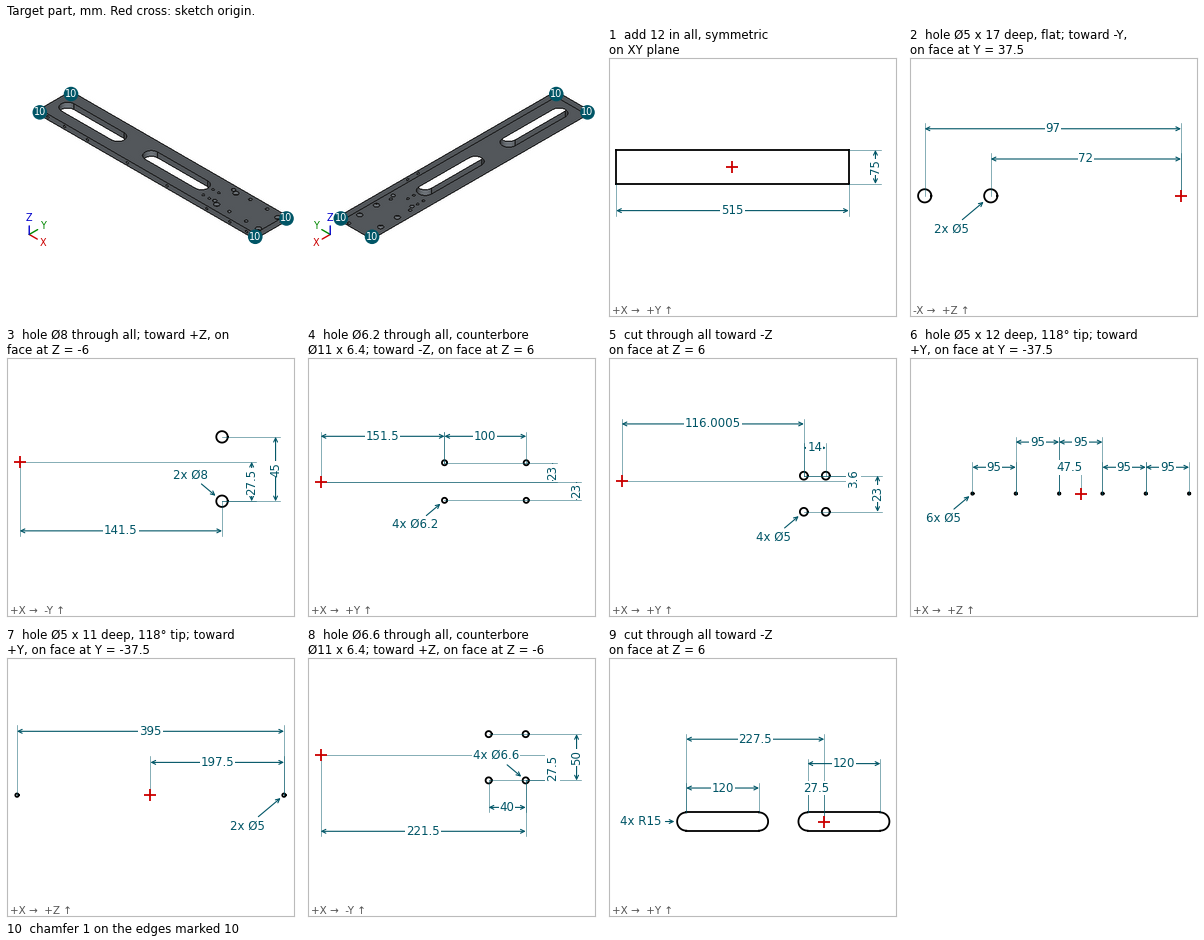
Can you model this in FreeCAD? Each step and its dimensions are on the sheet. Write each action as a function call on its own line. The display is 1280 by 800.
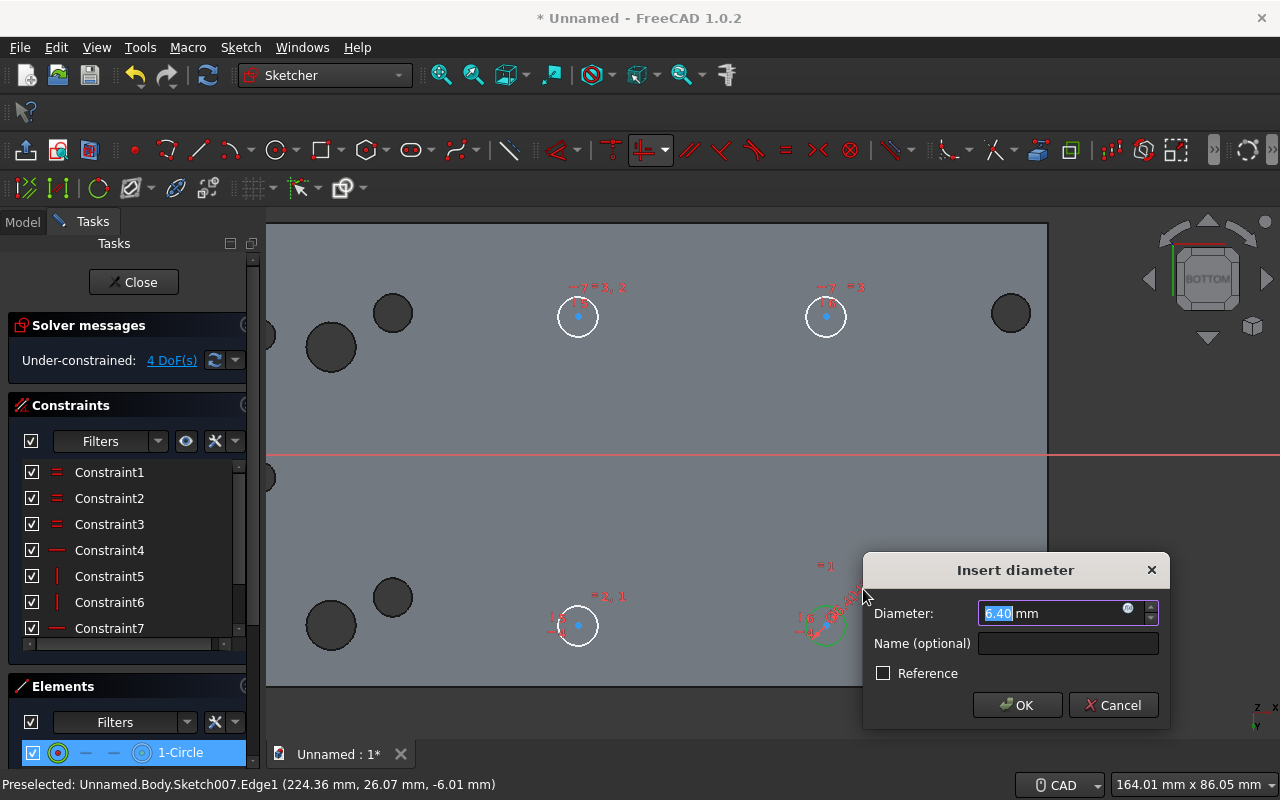
text(6.6)
key(Return)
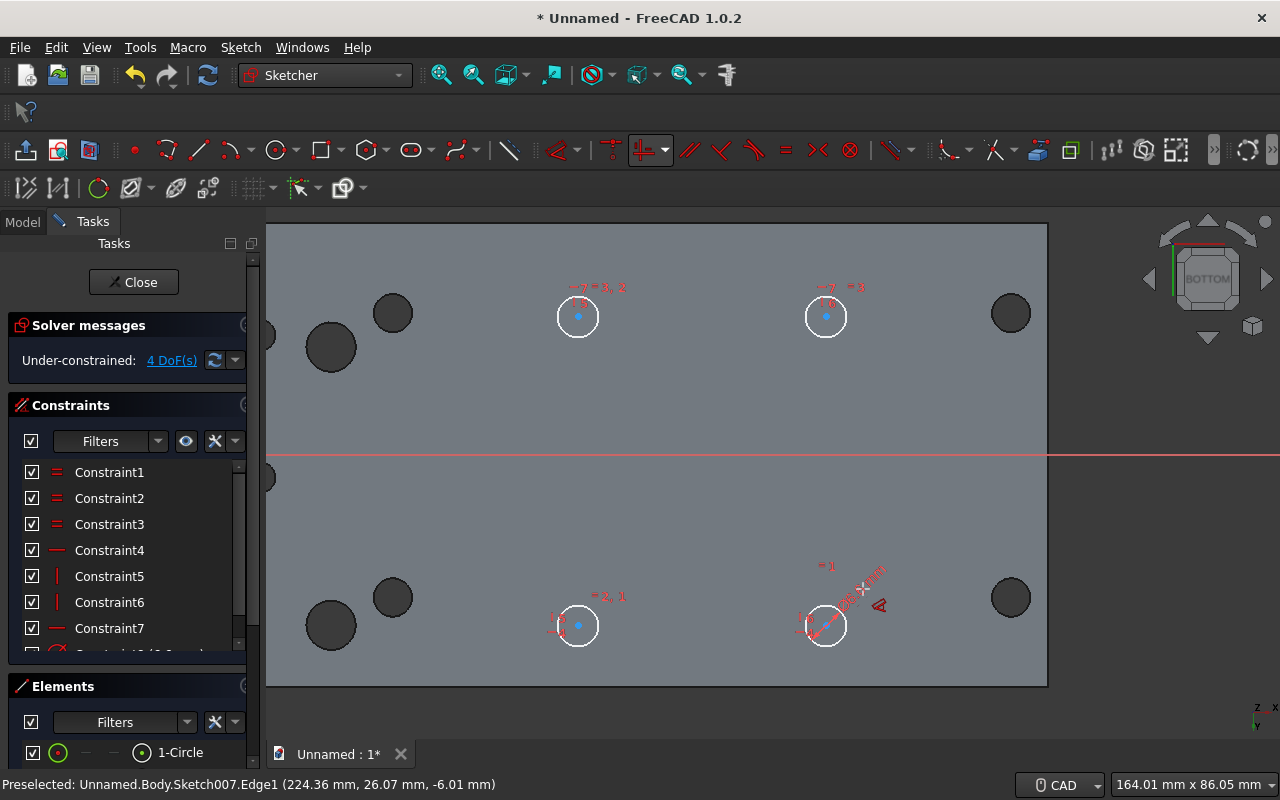
click(826, 626)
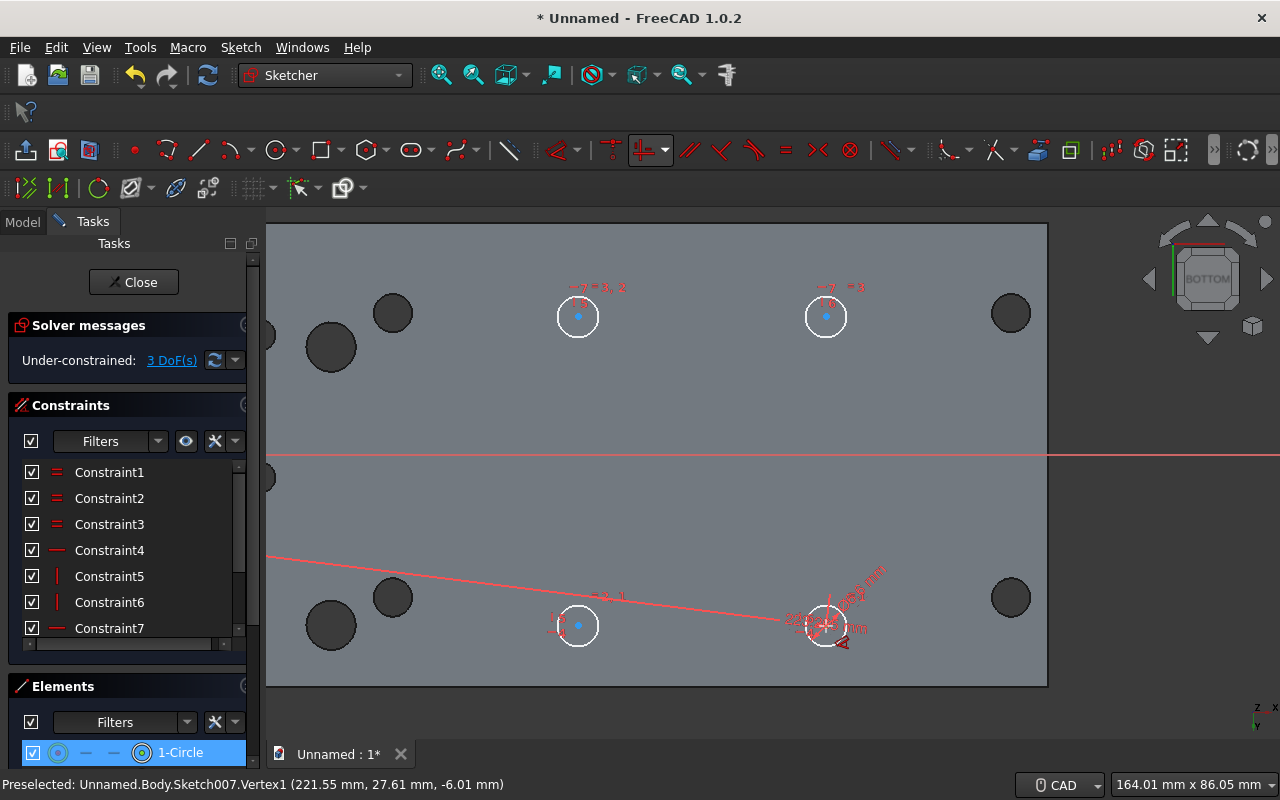
click(578, 626)
click(702, 660)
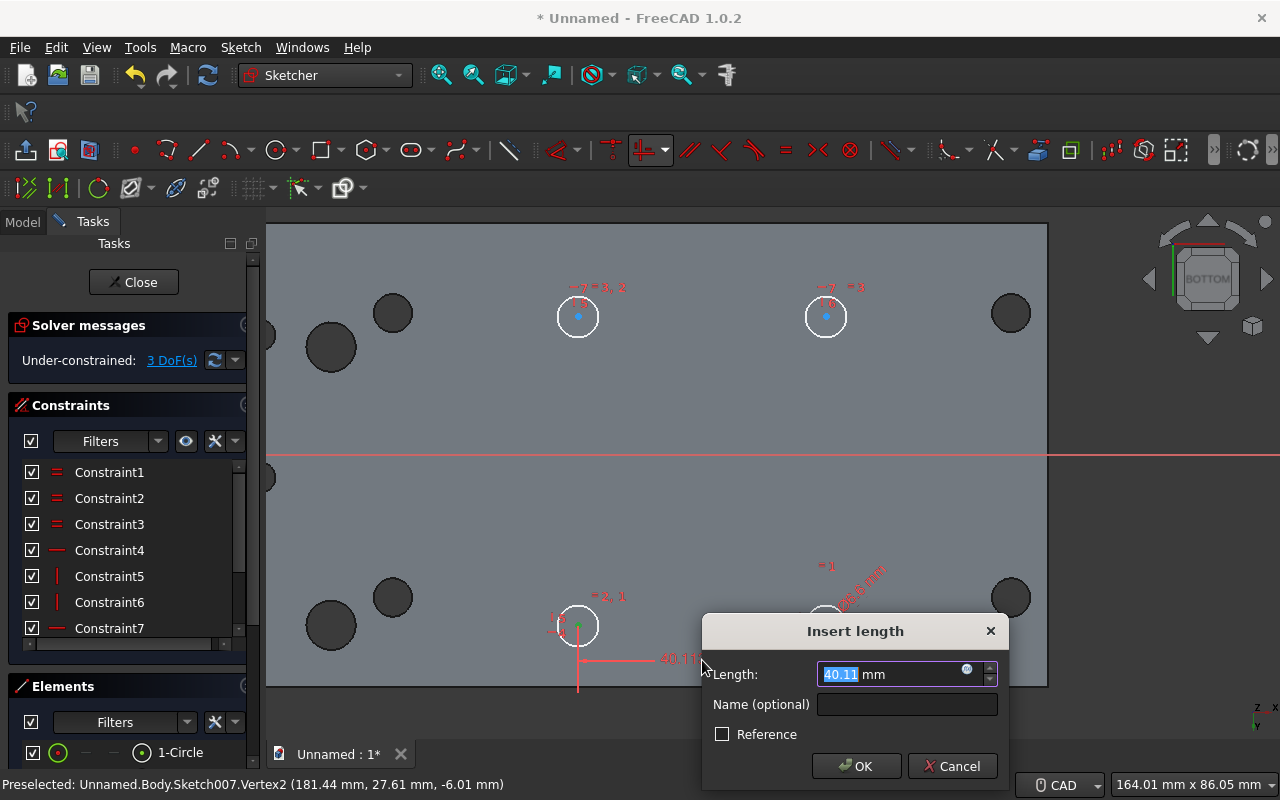
text(40)
key(Return)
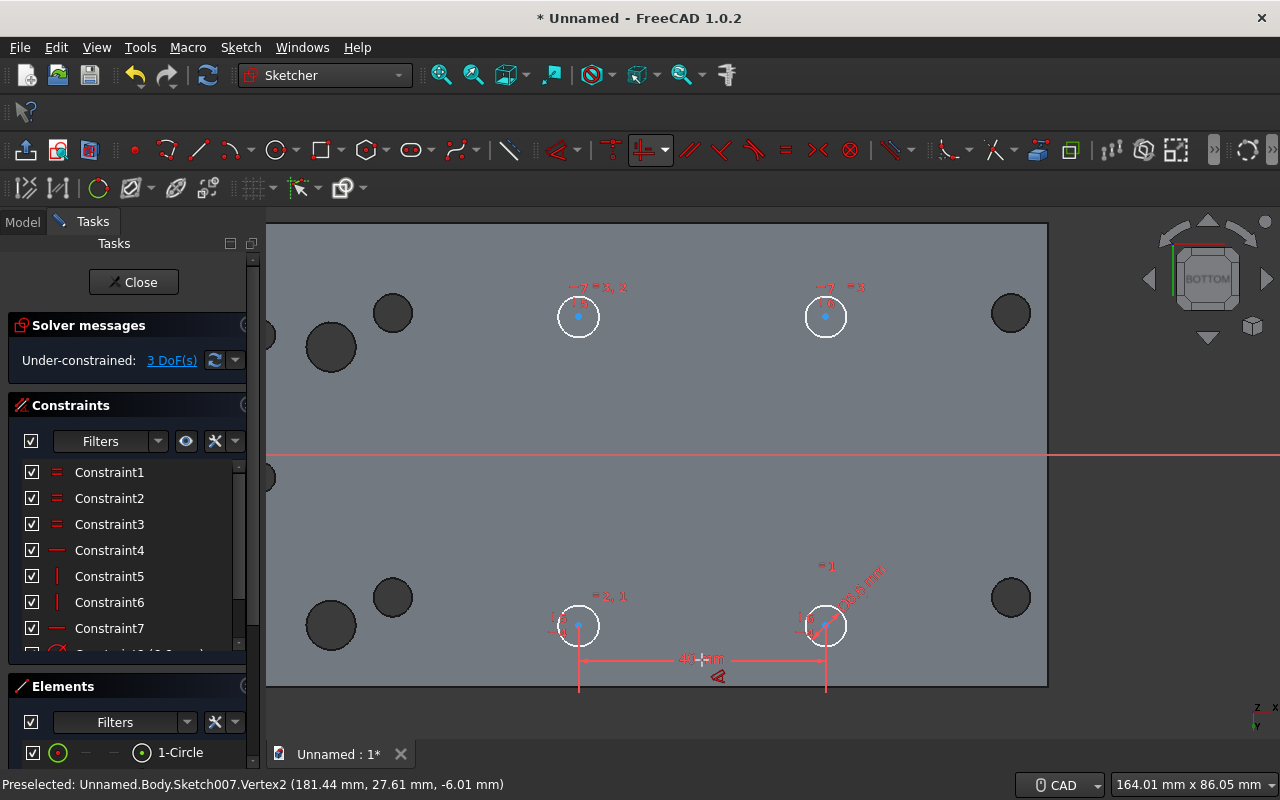
click(579, 626)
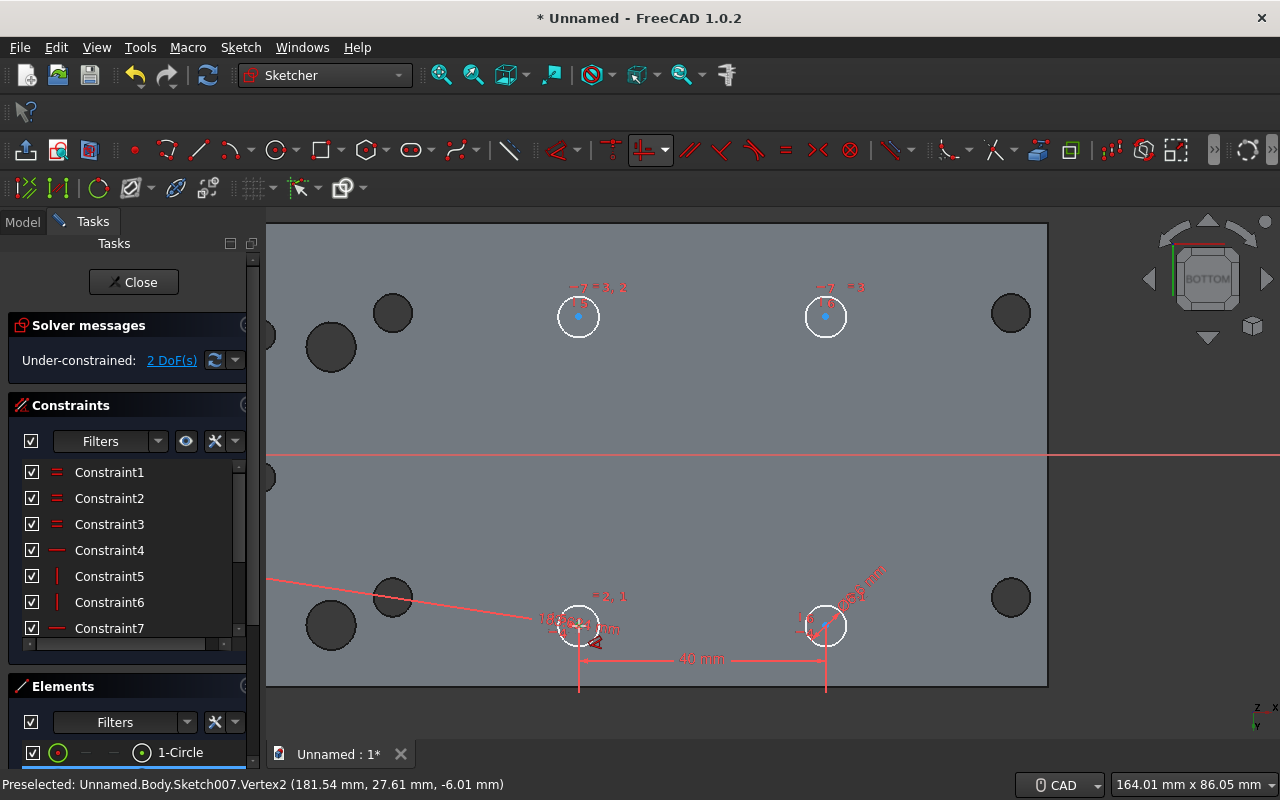
click(579, 317)
click(545, 471)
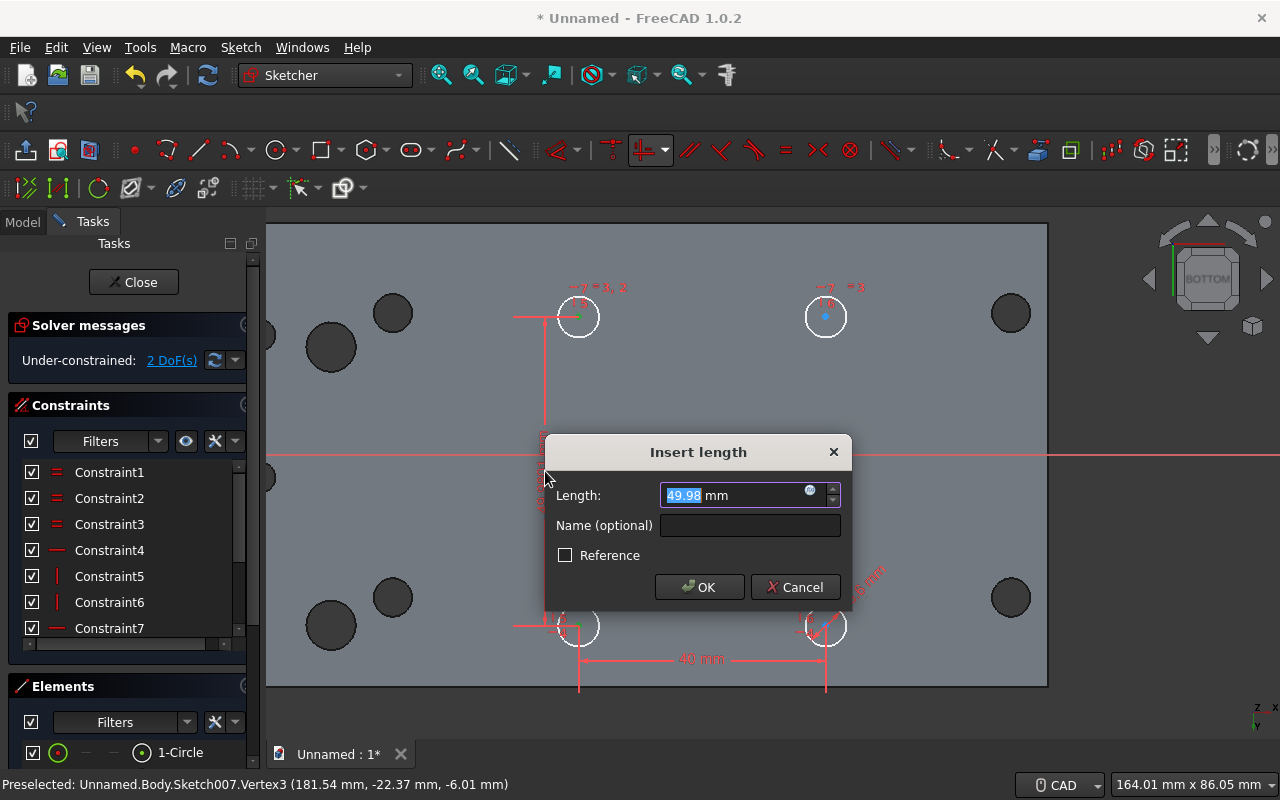
text(50)
key(Return)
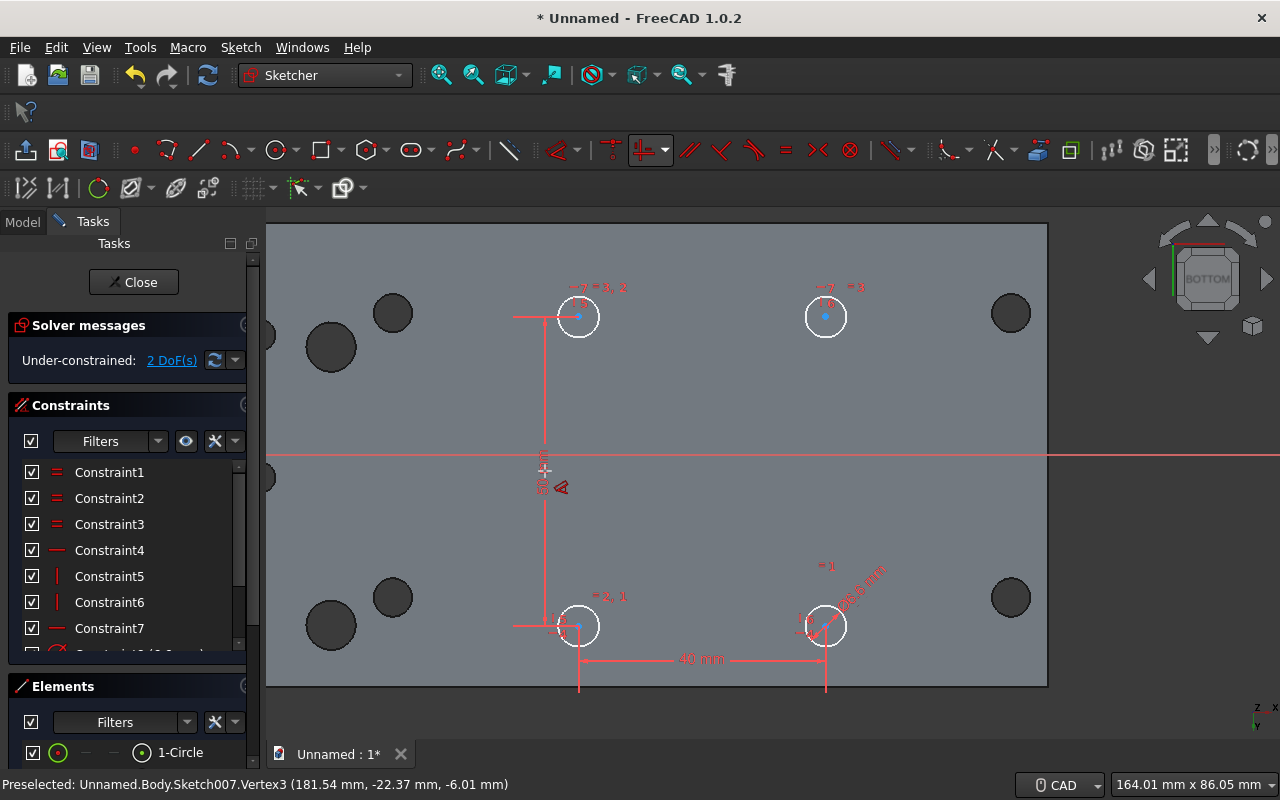
click(826, 626)
click(860, 541)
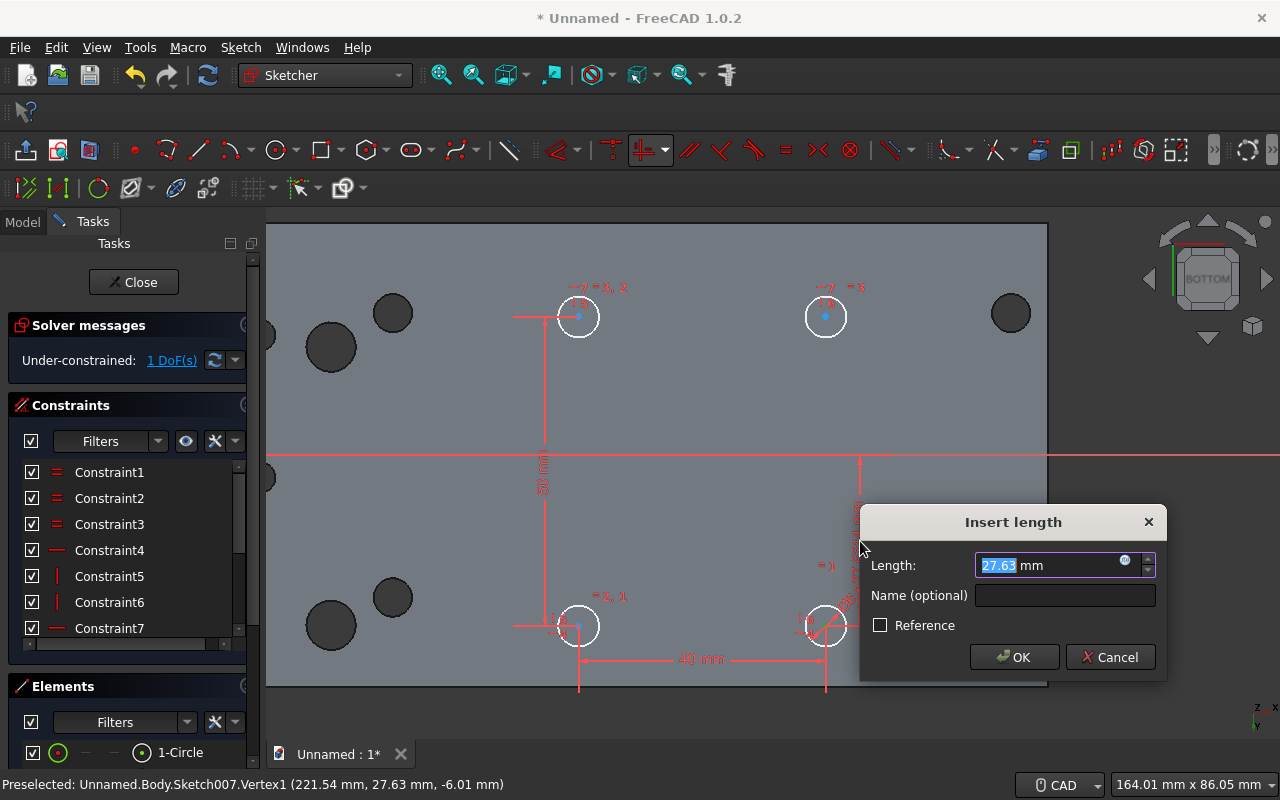
text(27.5)
key(Return)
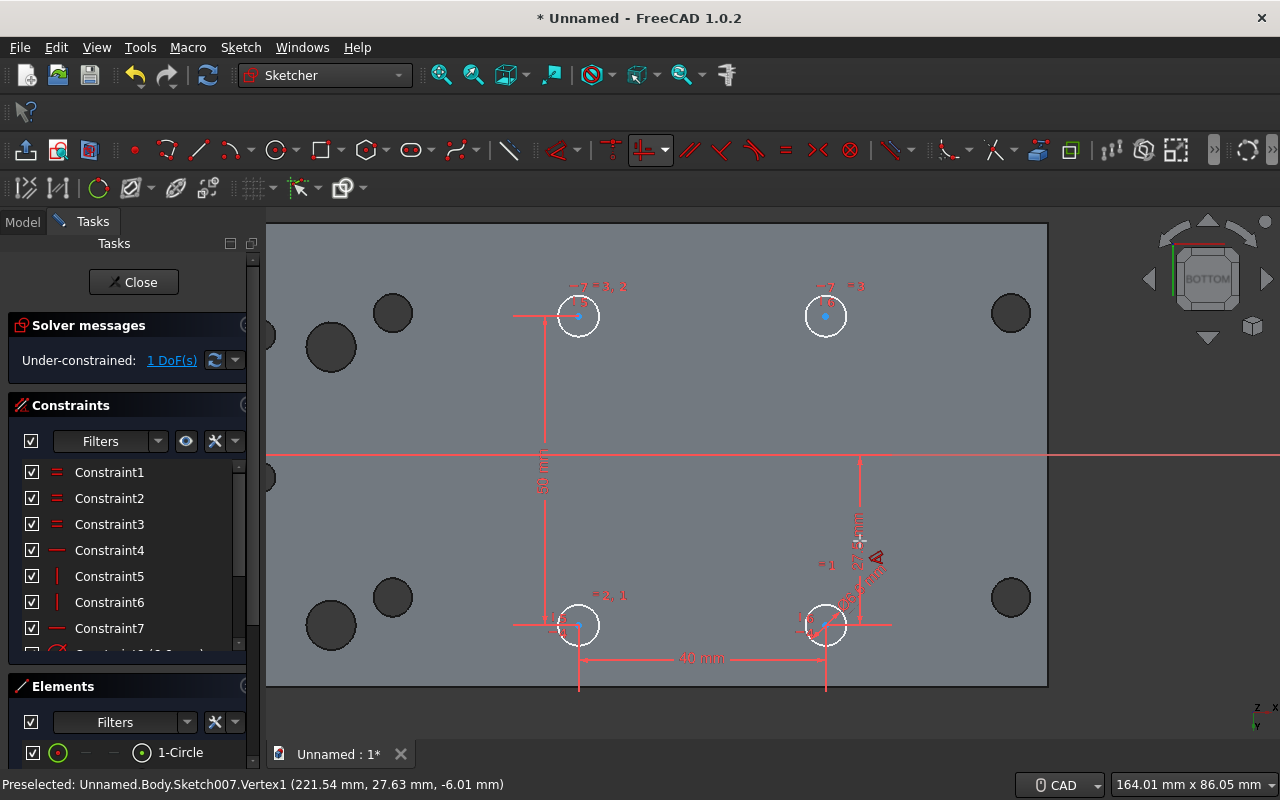
click(826, 625)
click(560, 659)